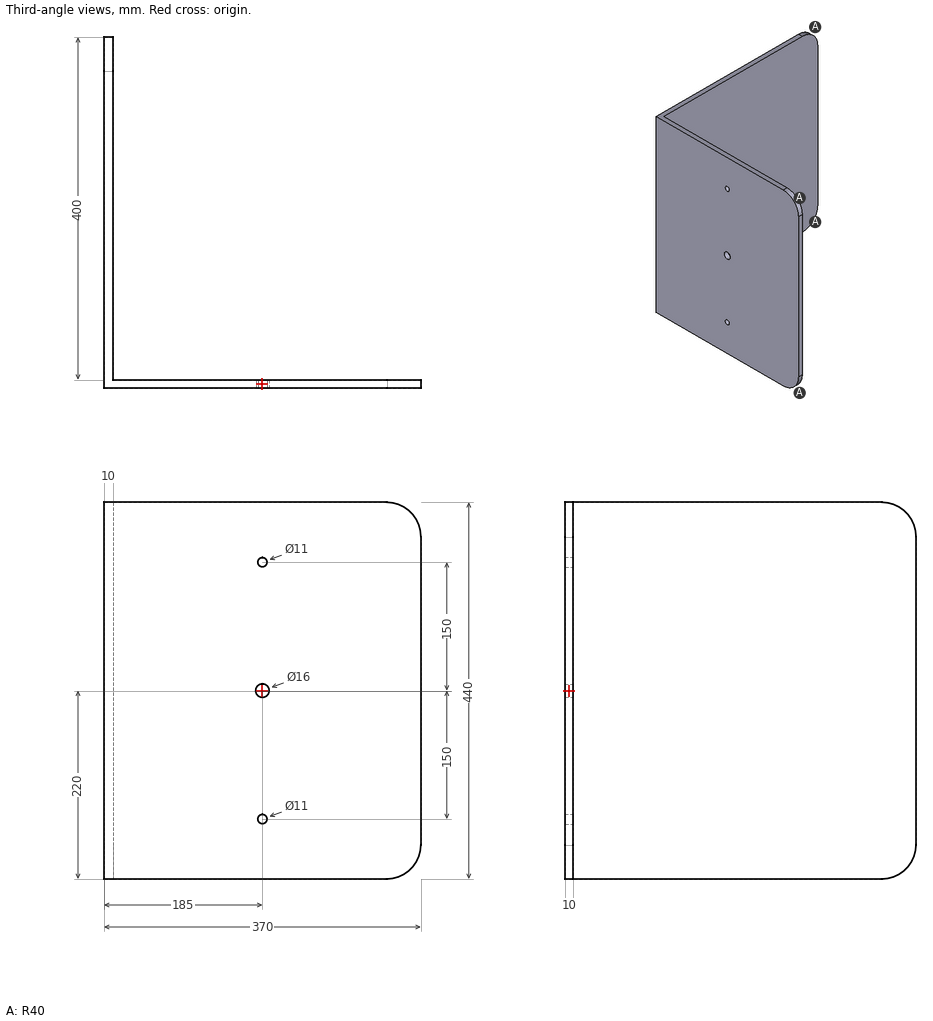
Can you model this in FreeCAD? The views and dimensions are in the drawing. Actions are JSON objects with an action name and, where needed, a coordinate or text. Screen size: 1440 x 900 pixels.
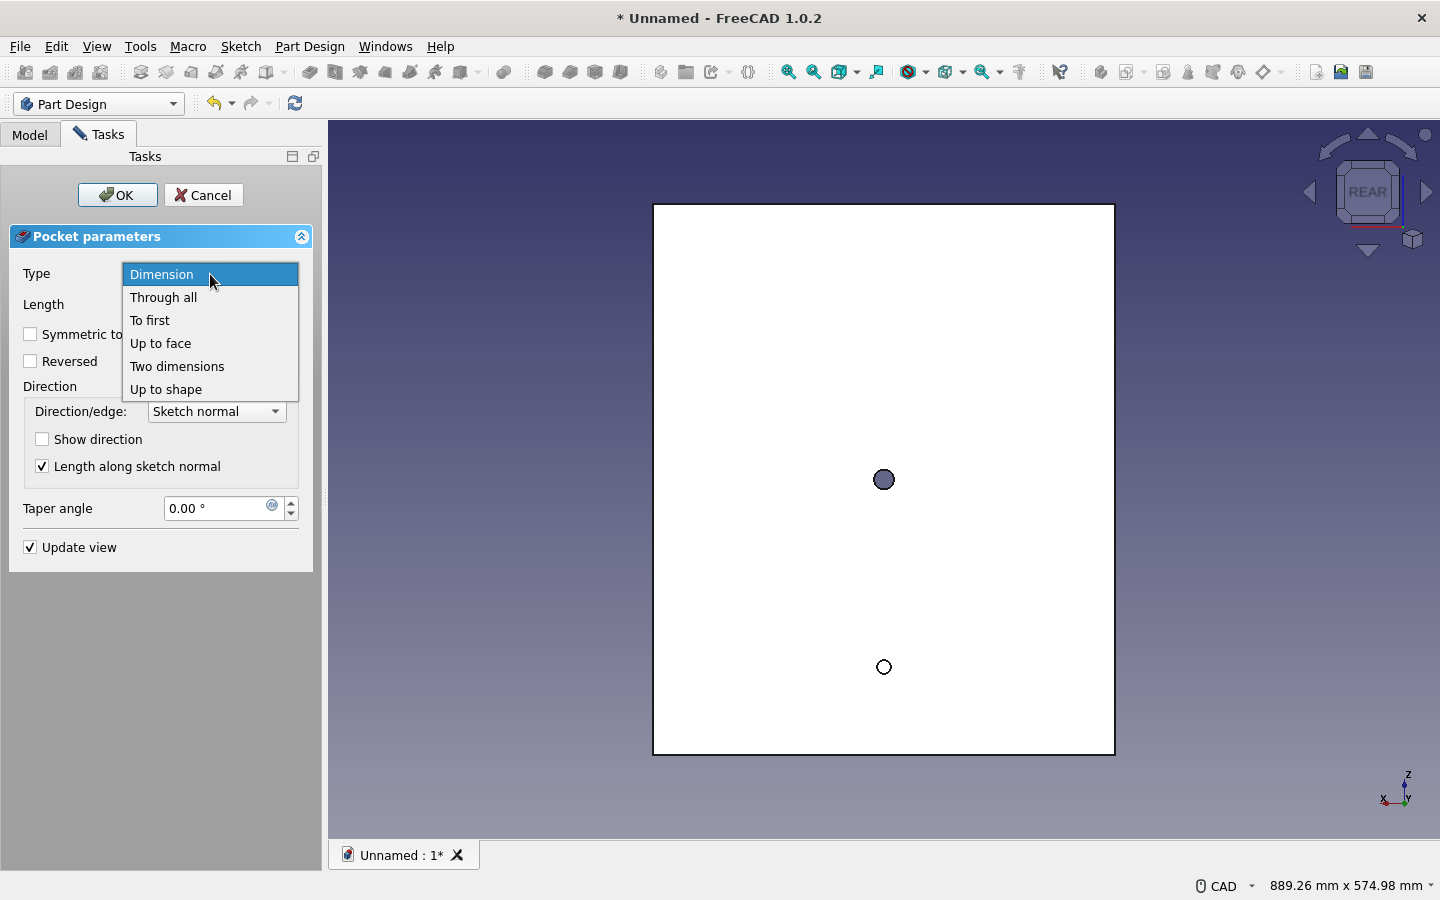
{"action": "left_click", "coordinate": [208, 320]}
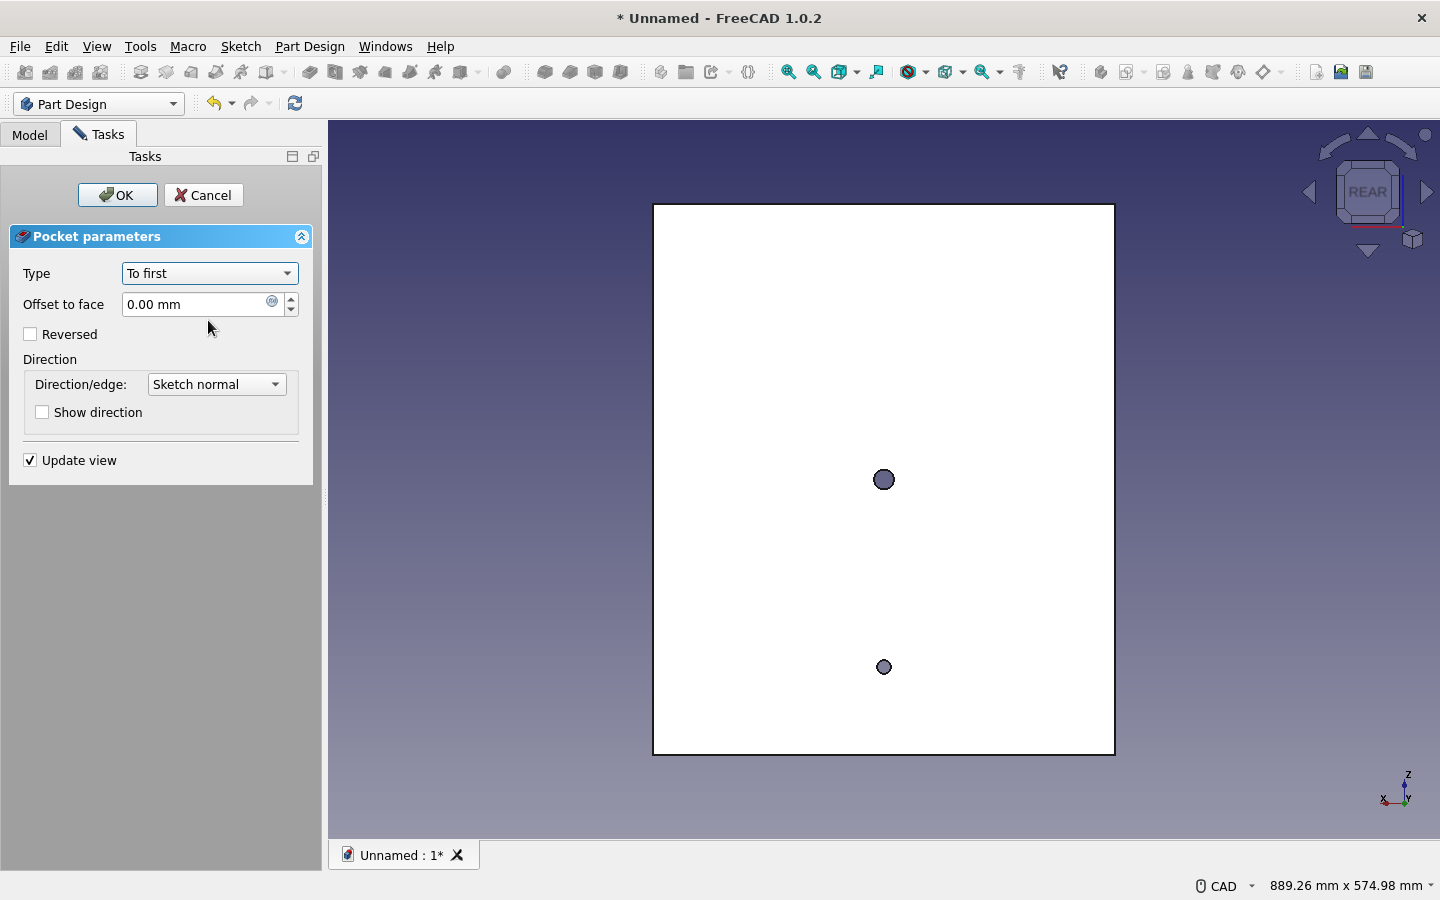
{"action": "left_click", "coordinate": [118, 195]}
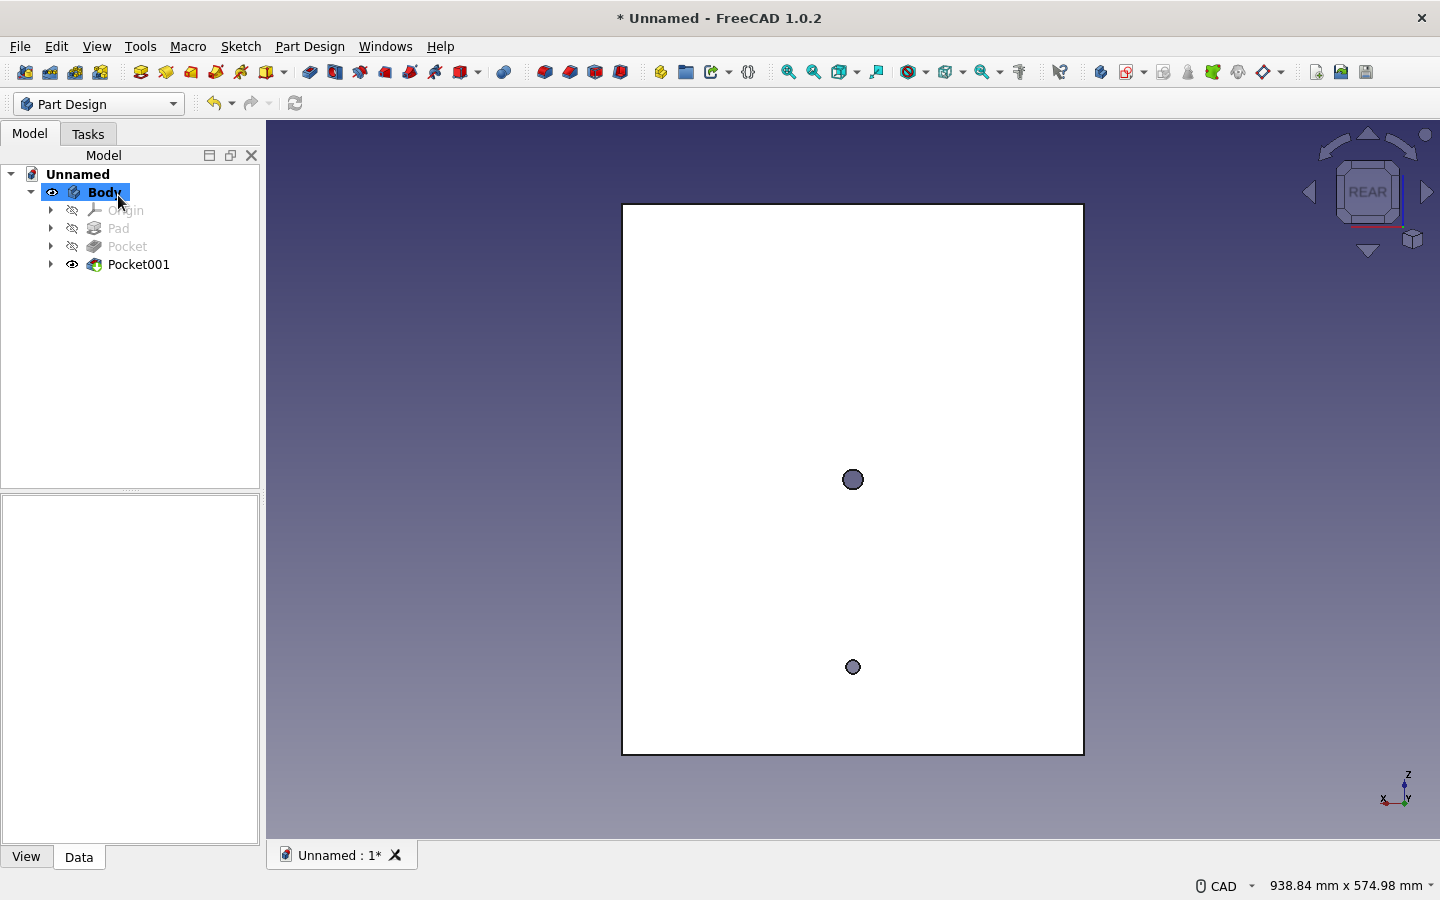
{"action": "left_click", "coordinate": [787, 321]}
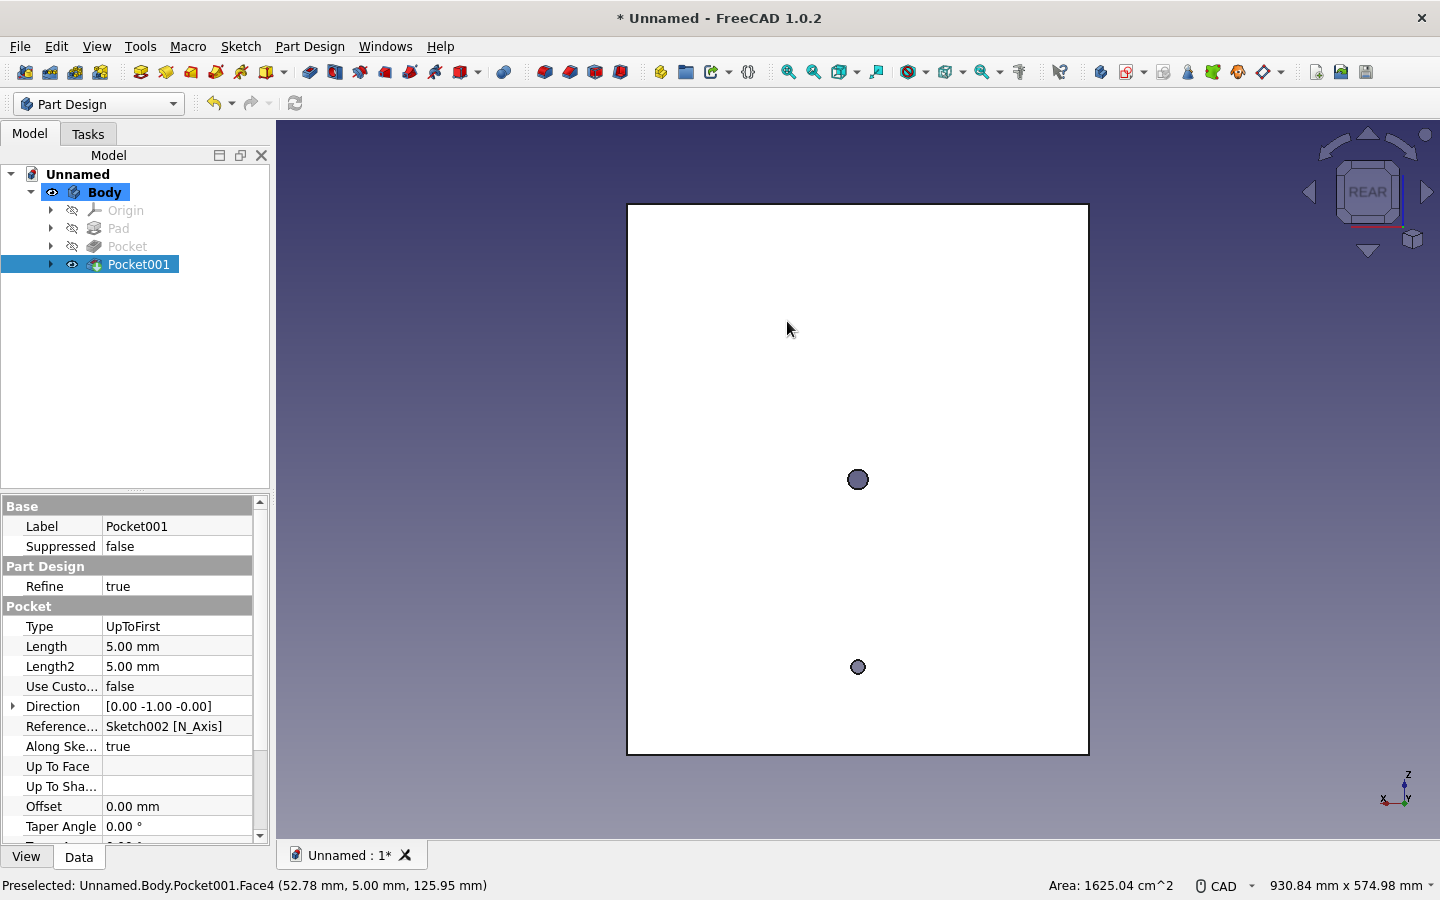
{"action": "left_click", "coordinate": [1126, 72]}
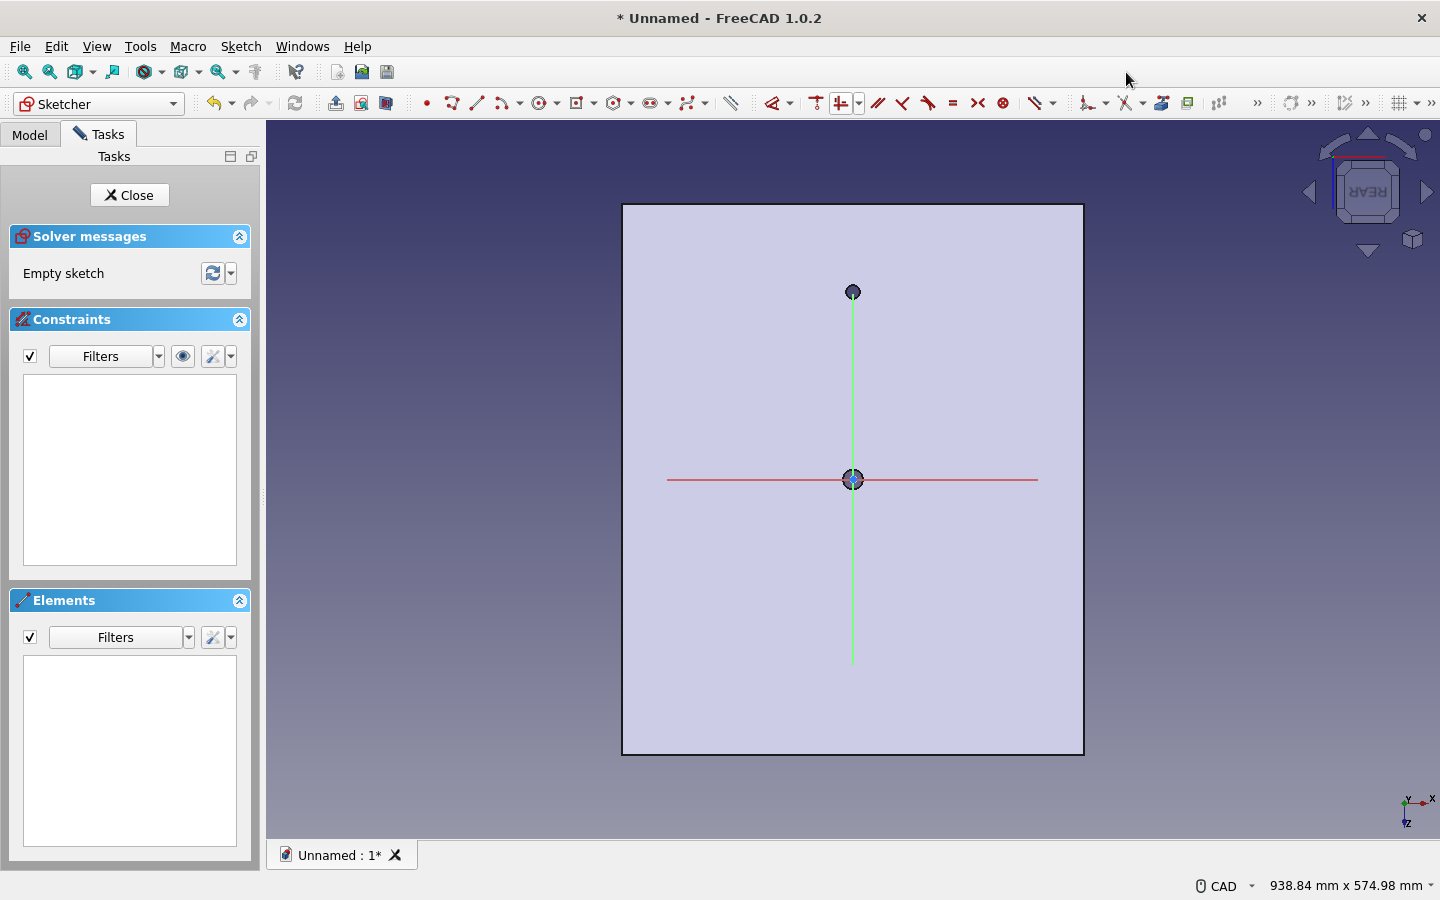
{"action": "scroll", "coordinate": [857, 677], "scroll_direction": "up", "scroll_amount": 15}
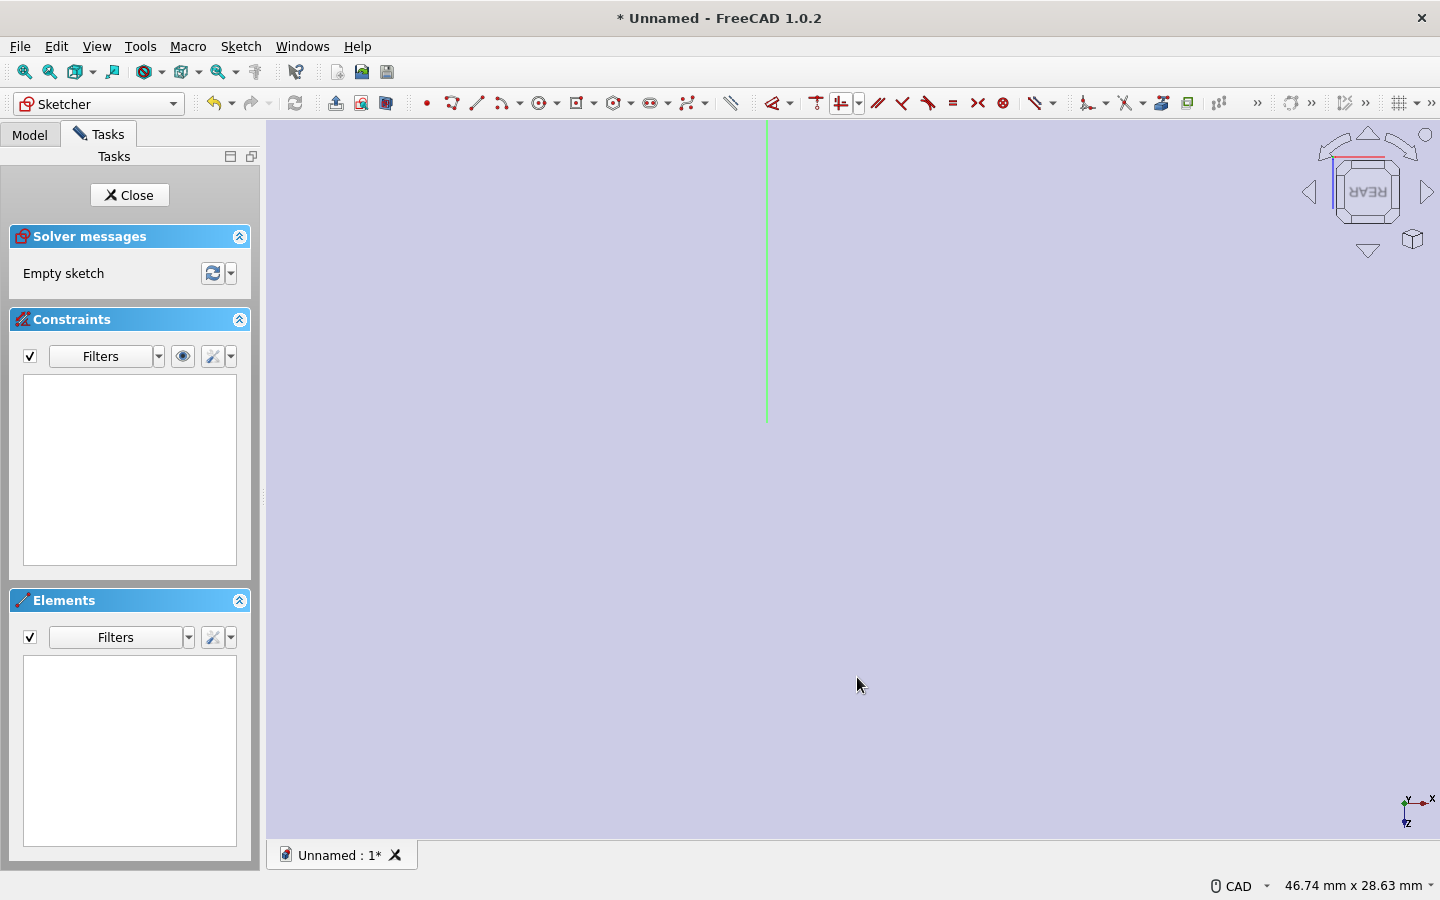
{"action": "scroll", "coordinate": [746, 442], "scroll_direction": "up", "scroll_amount": 3}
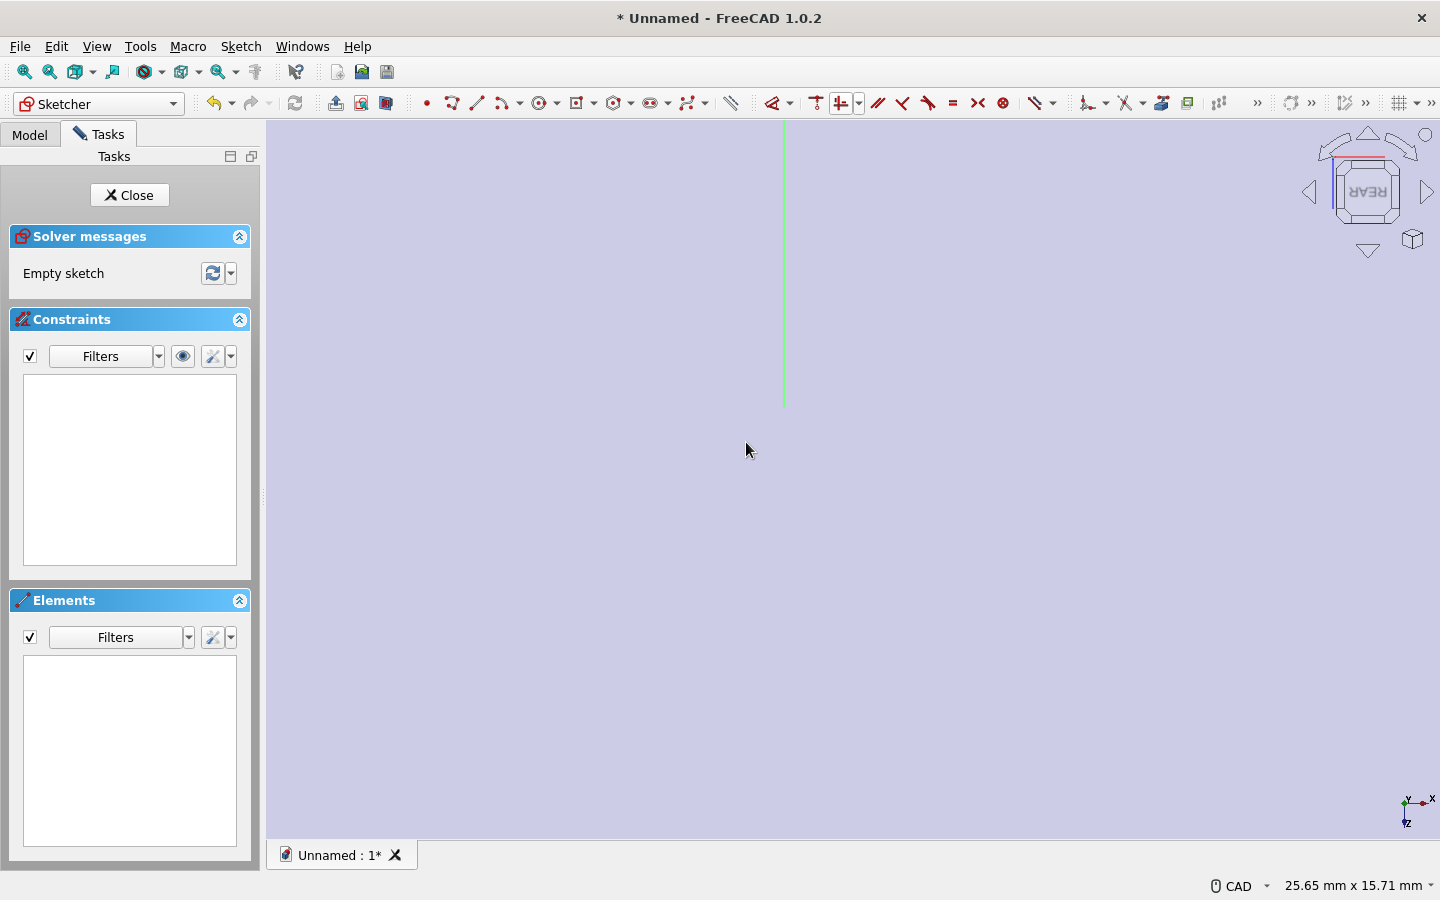
{"action": "left_click", "coordinate": [538, 104]}